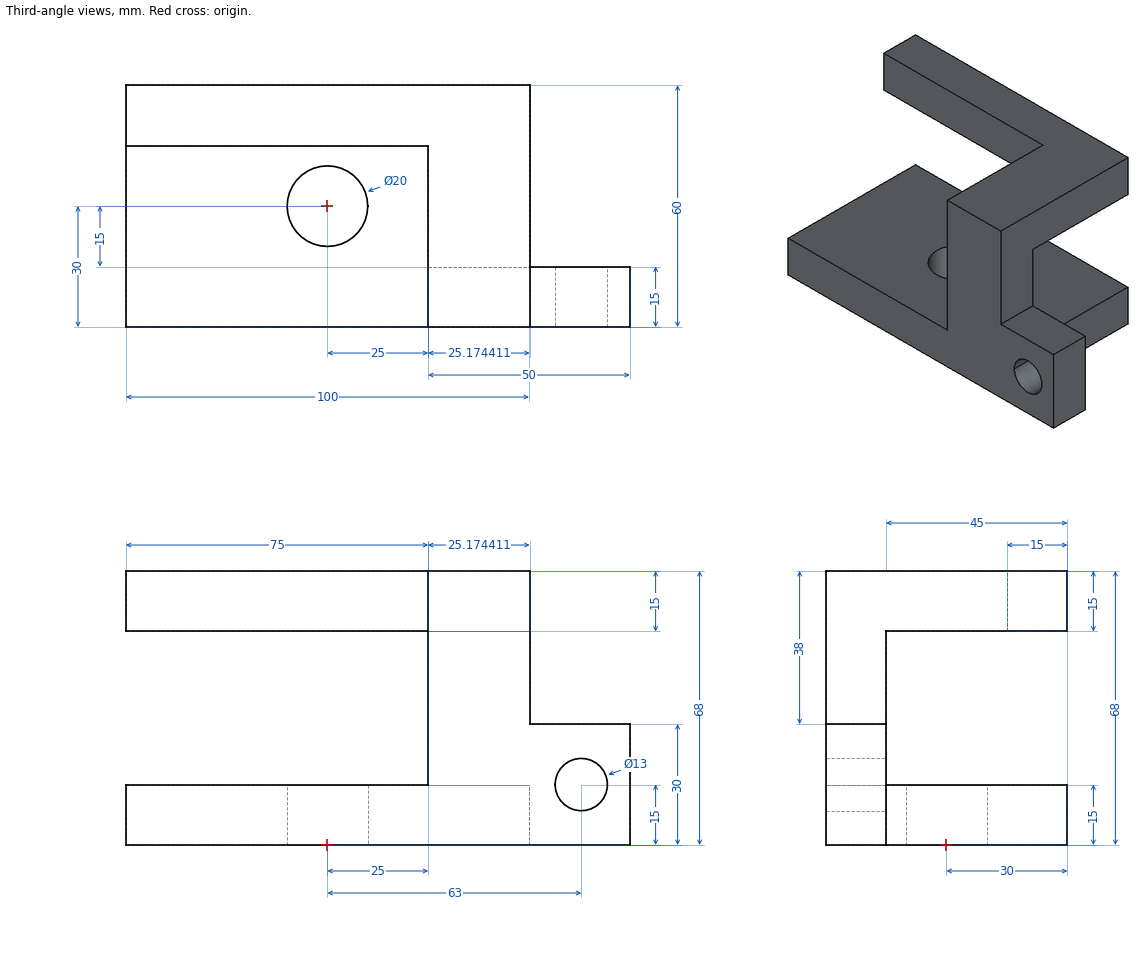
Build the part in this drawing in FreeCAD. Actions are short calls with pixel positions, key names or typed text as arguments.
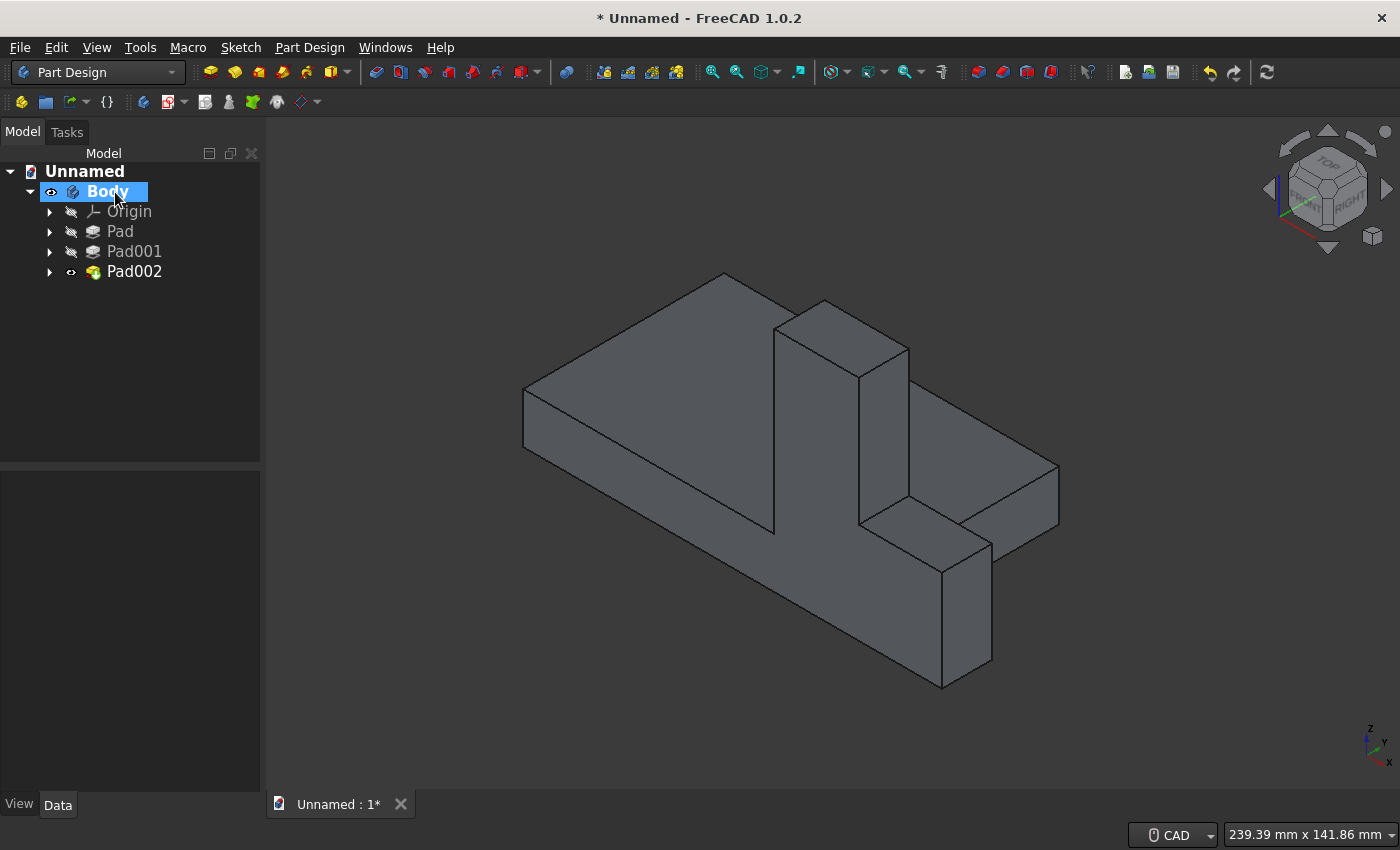
click(714, 72)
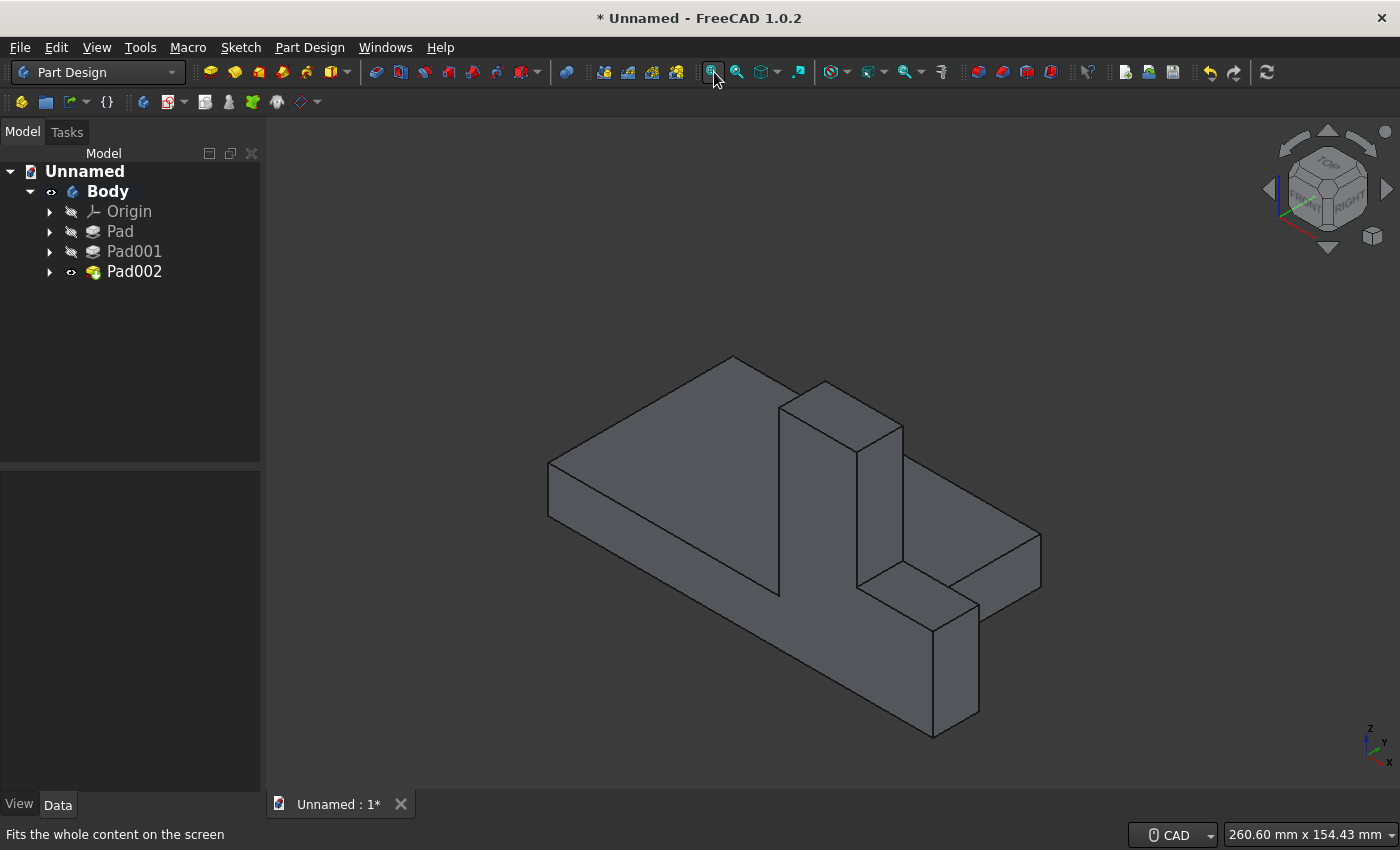
key(4)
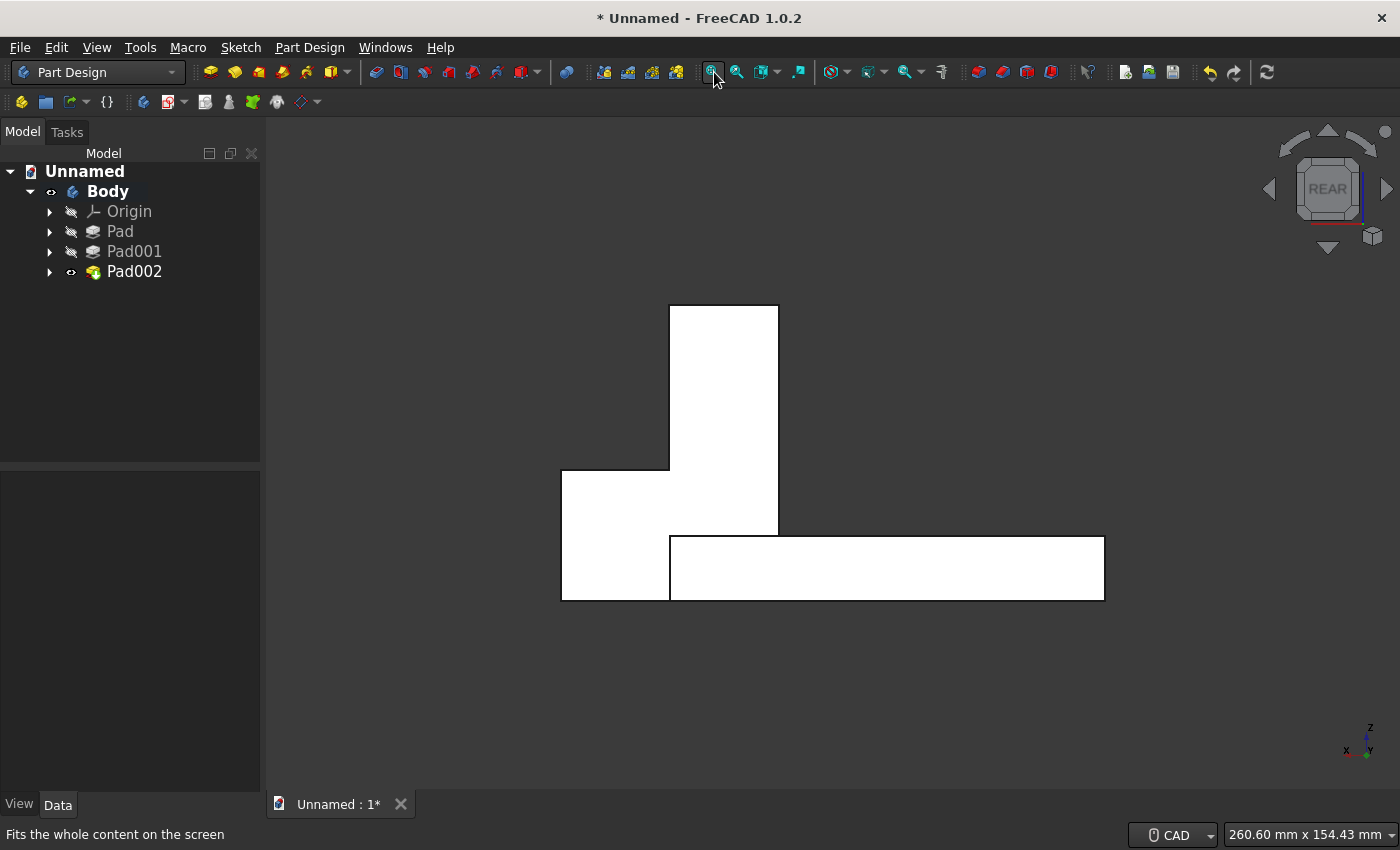
click(608, 537)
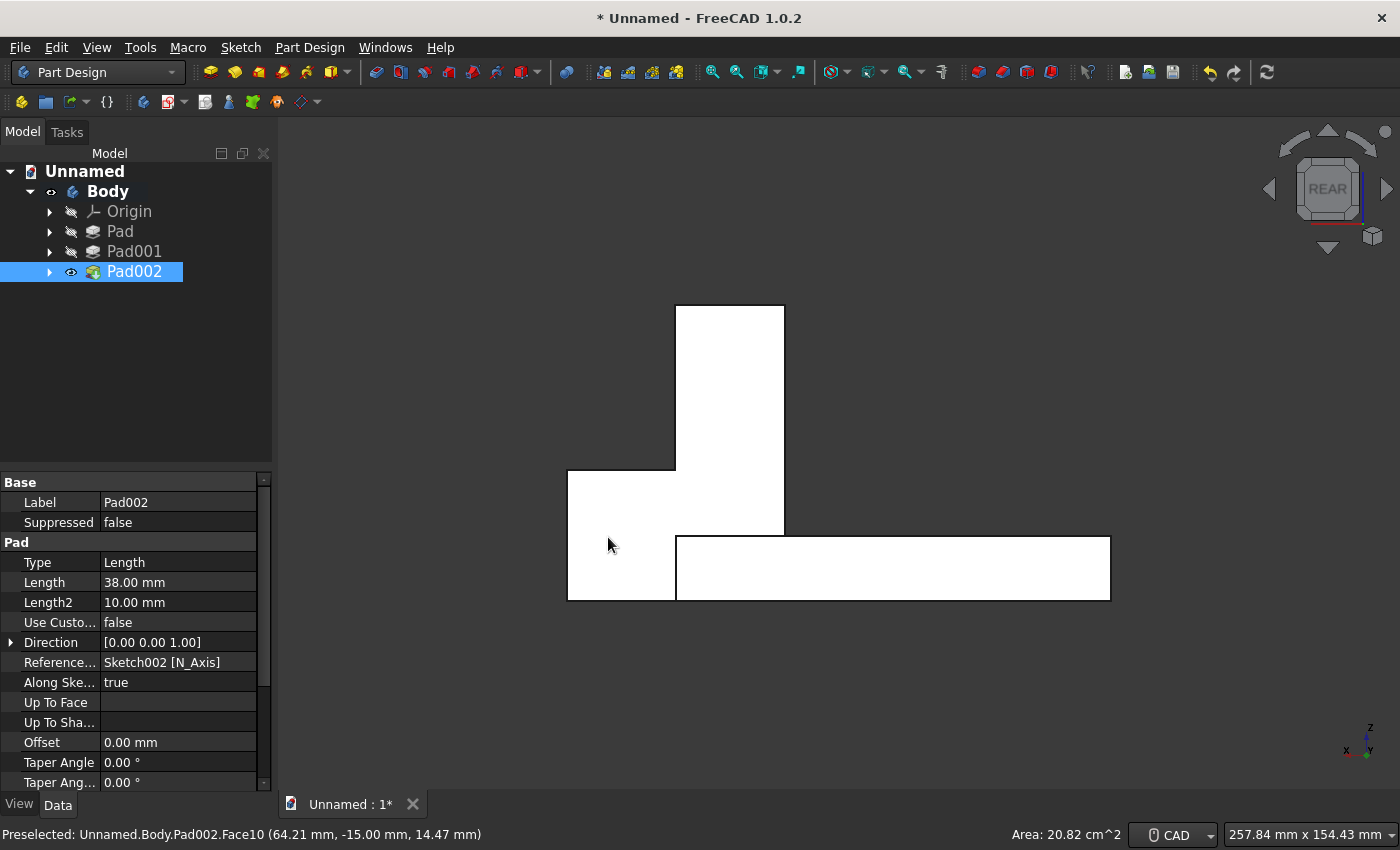
click(168, 102)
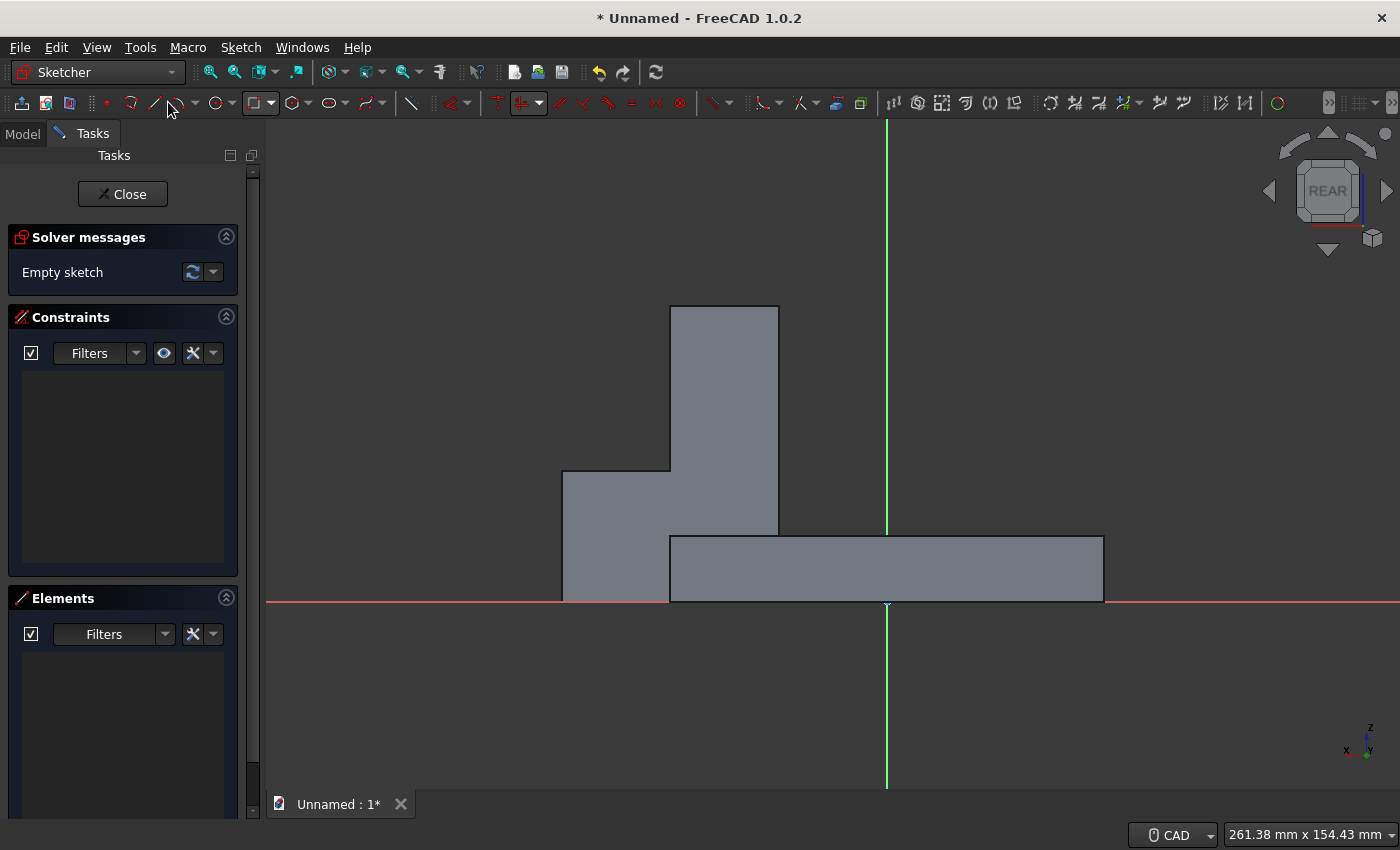
scroll(716, 316, up, 9)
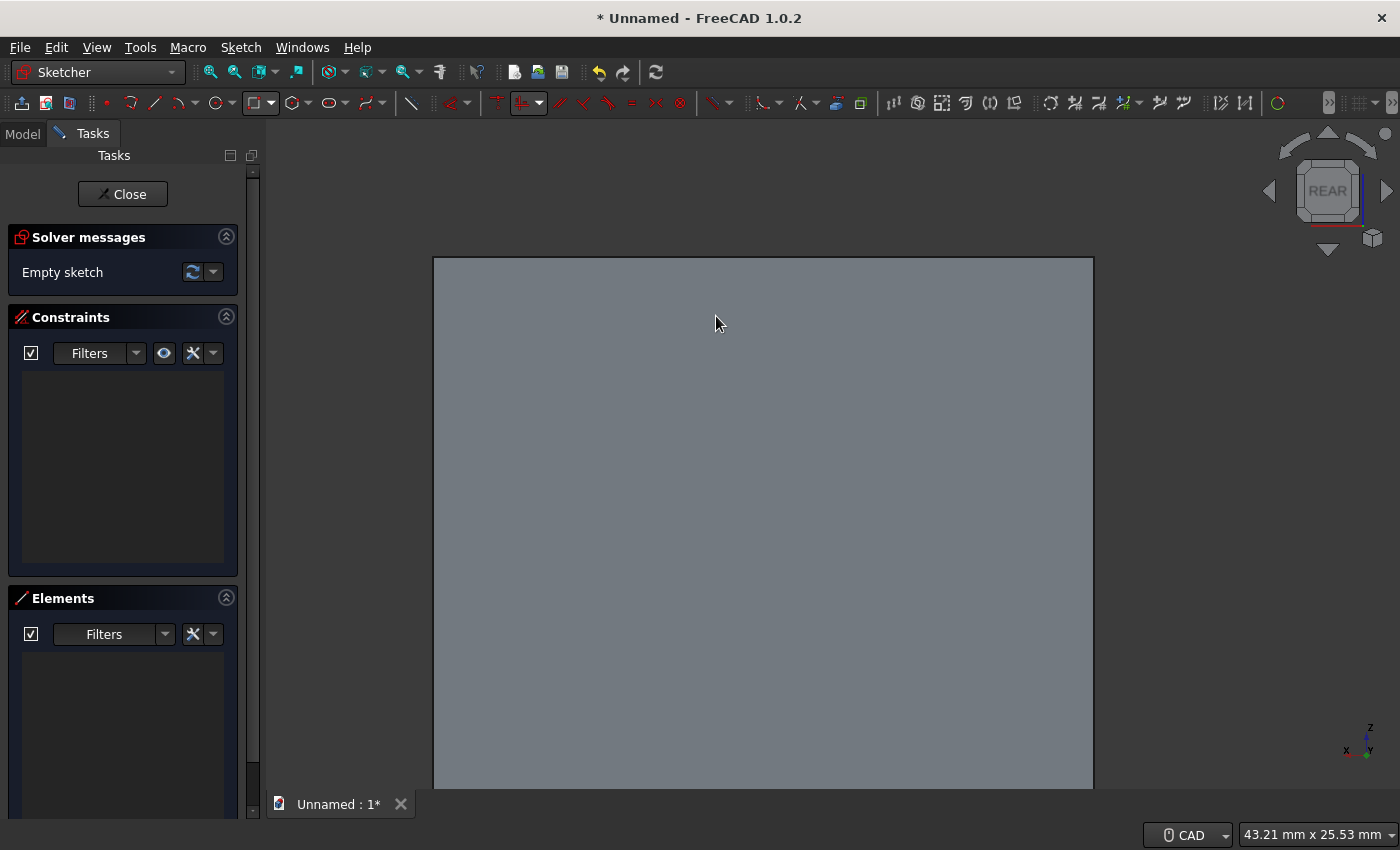
click(254, 104)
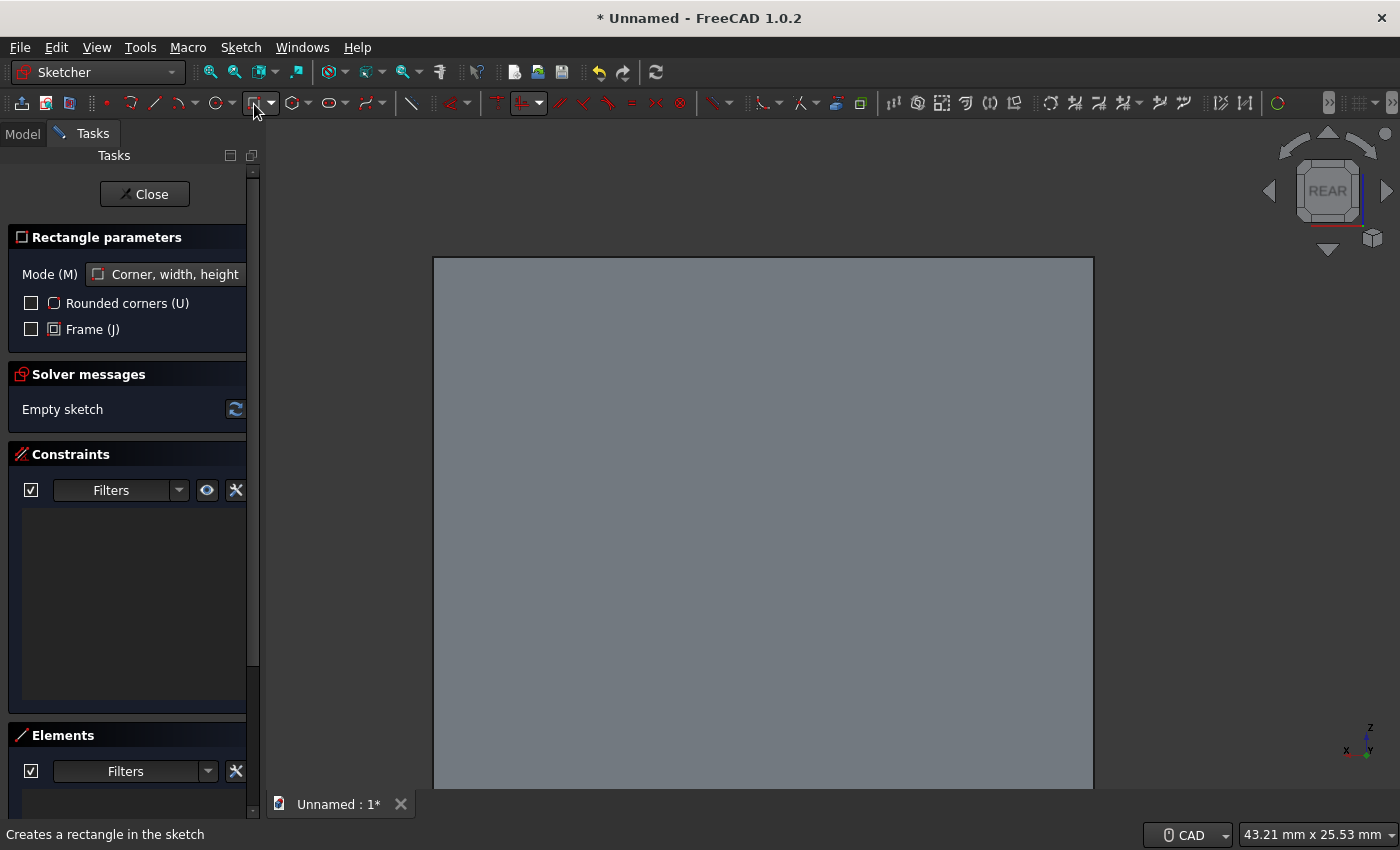
click(433, 257)
move(1094, 651)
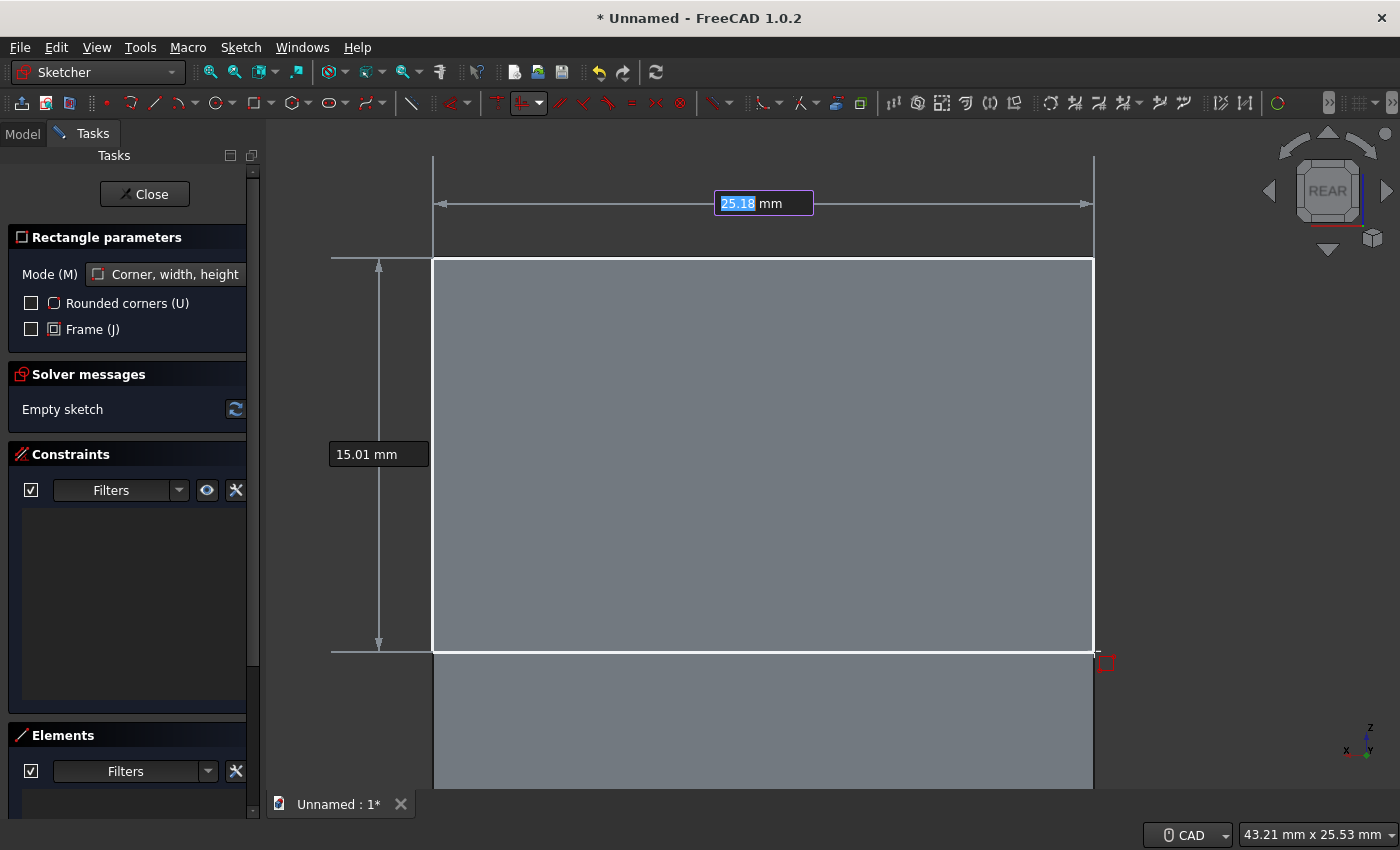
text(25.174411)
key(Tab)
text(15)
key(Return)
key(Escape)